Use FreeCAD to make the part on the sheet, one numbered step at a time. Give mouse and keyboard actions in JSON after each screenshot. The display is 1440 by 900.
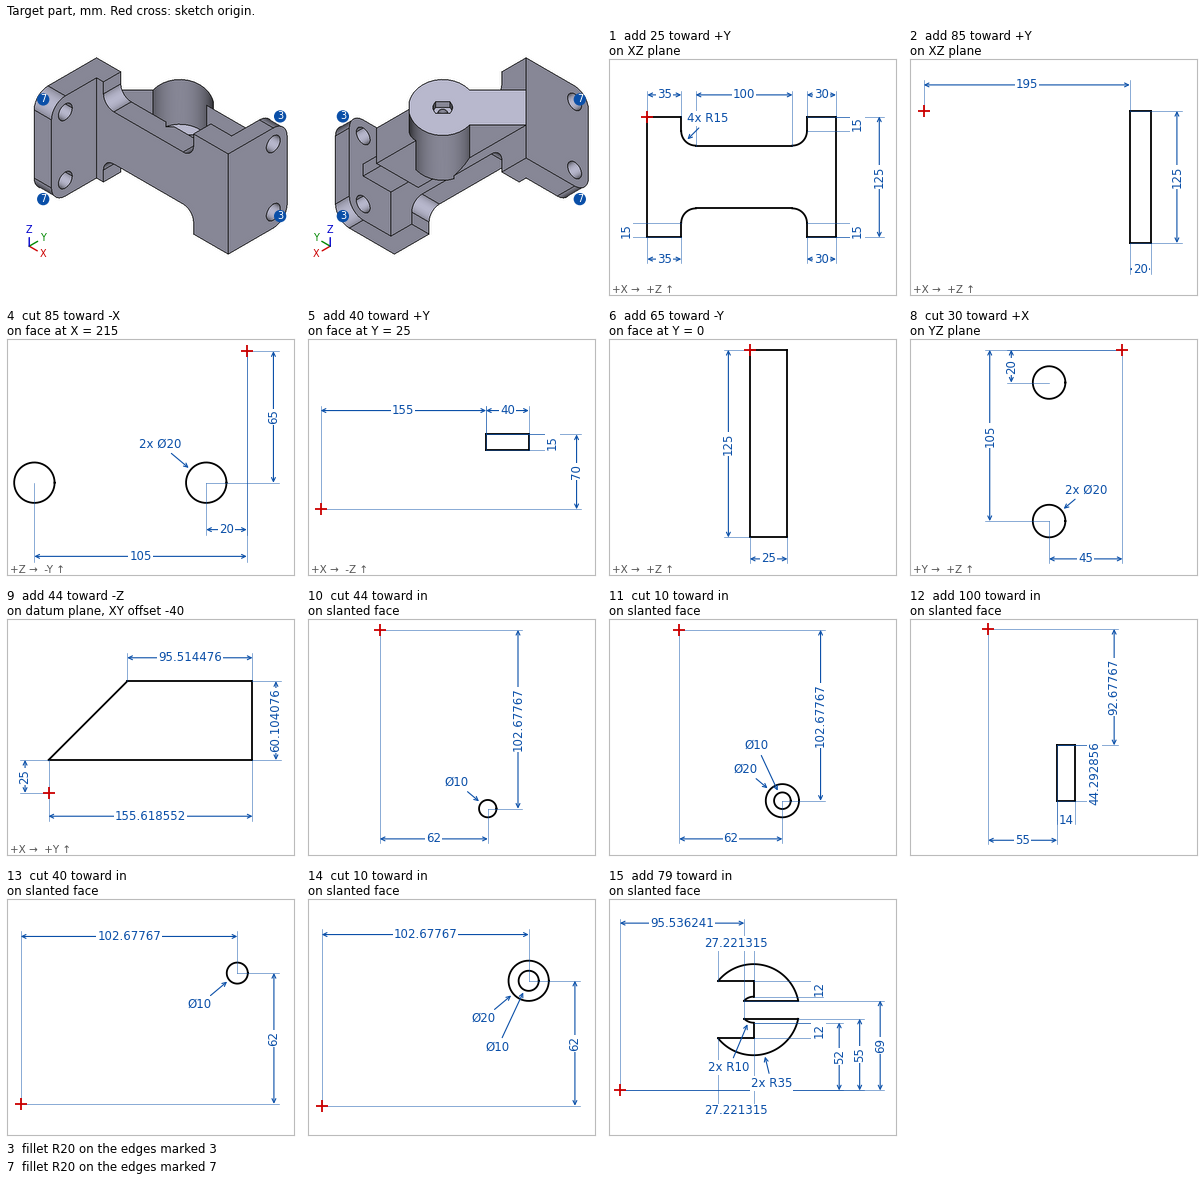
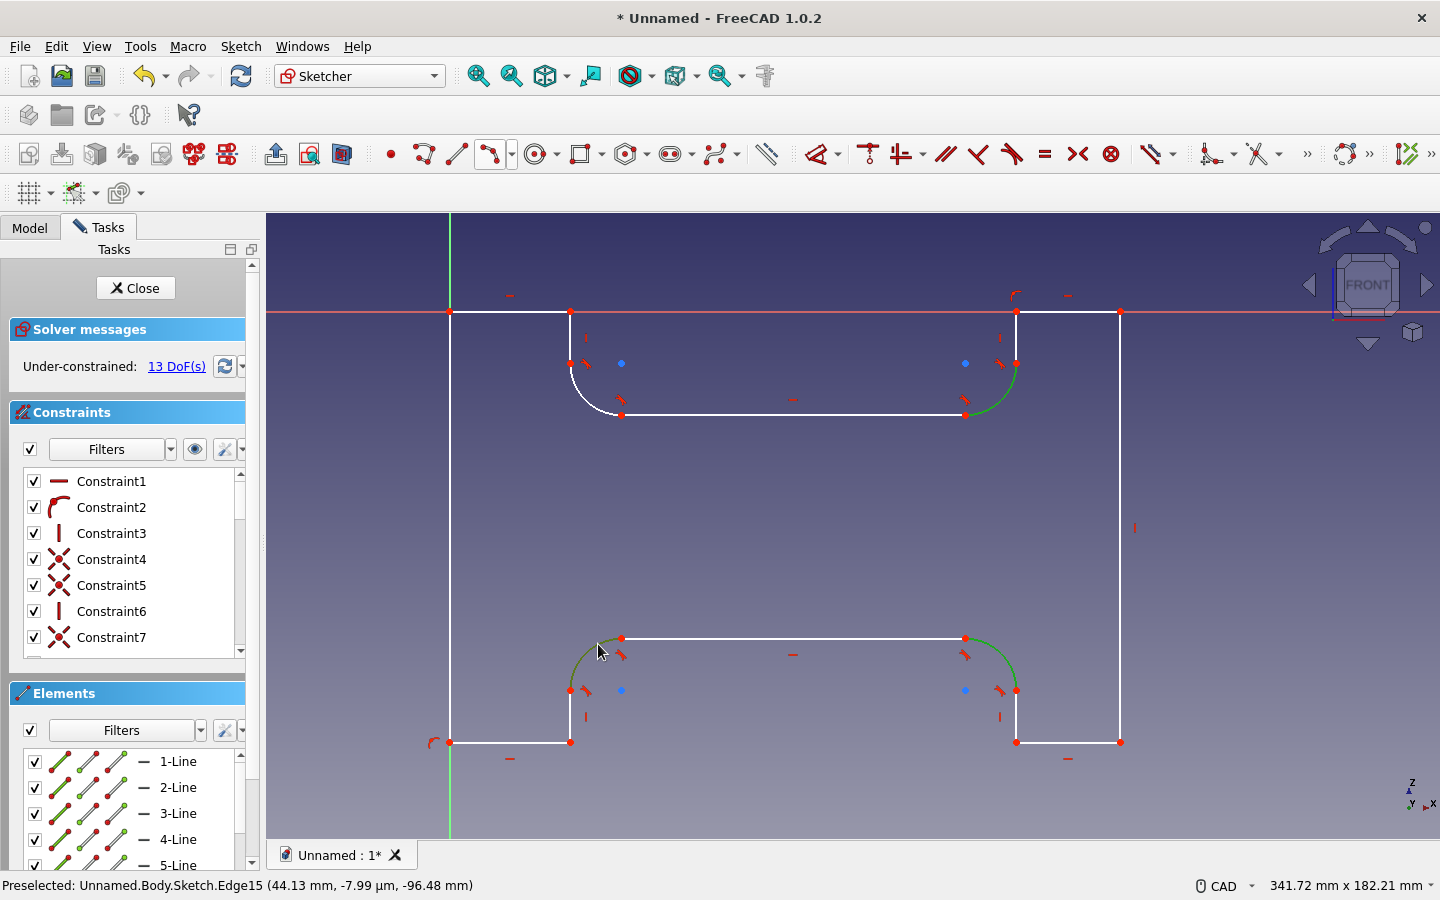
{"action": "left_click", "coordinate": [576, 387]}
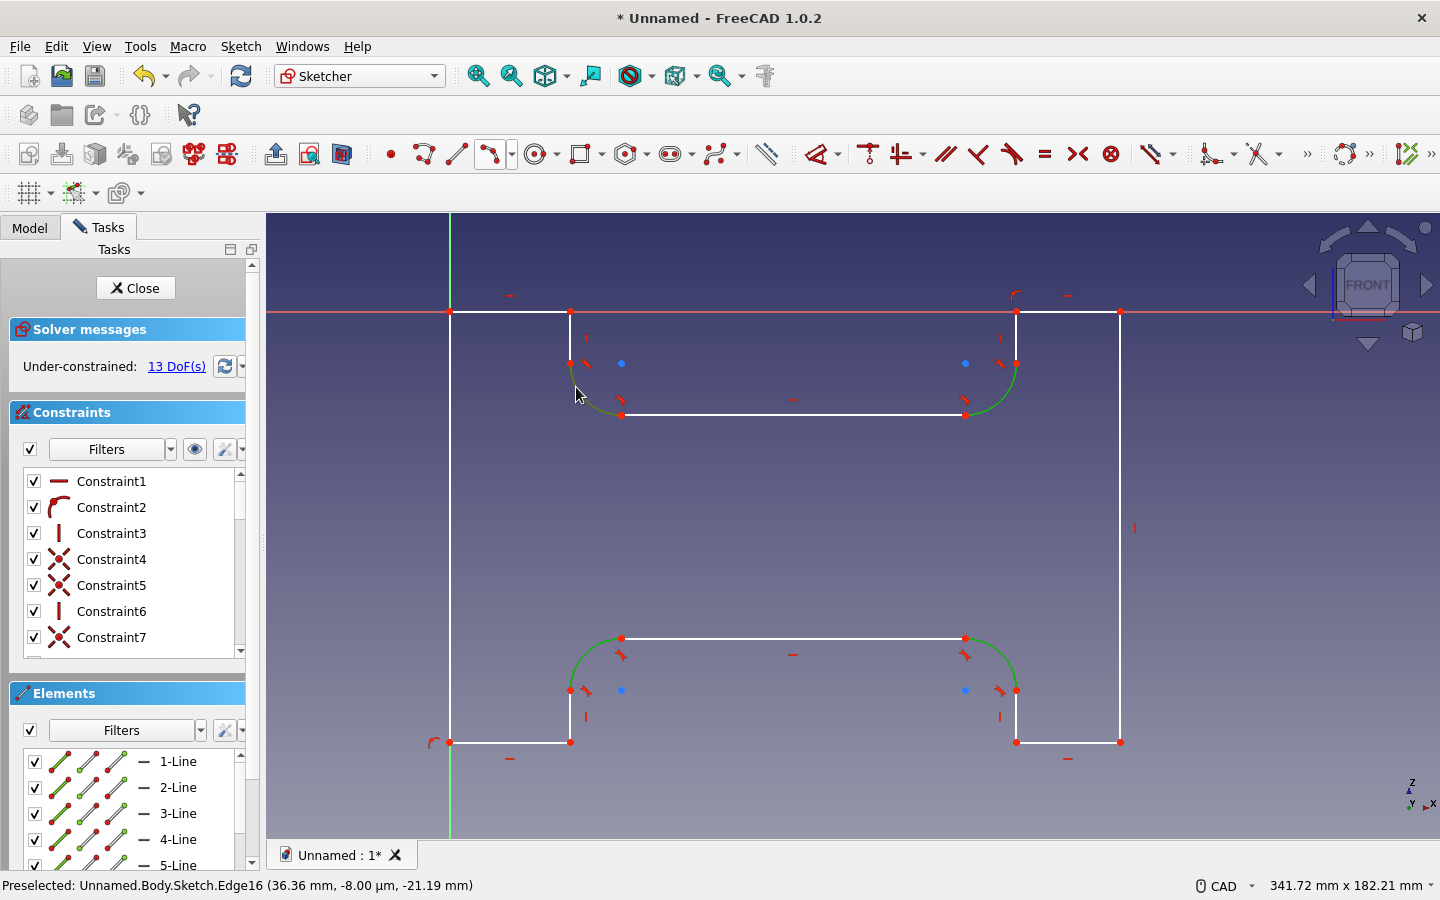
{"action": "key", "text": "e"}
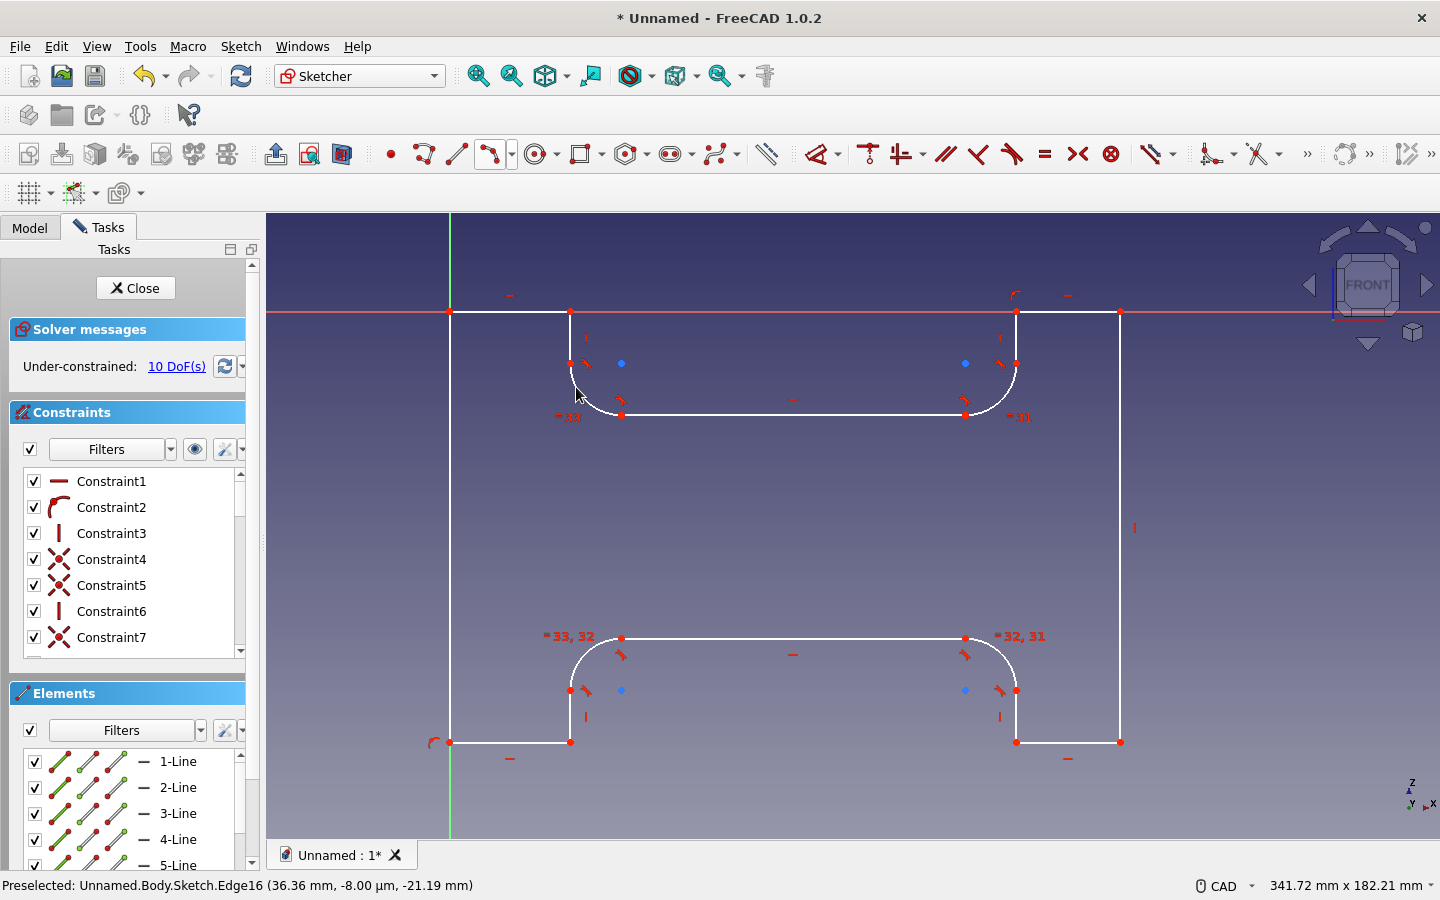
{"action": "left_click", "coordinate": [816, 154]}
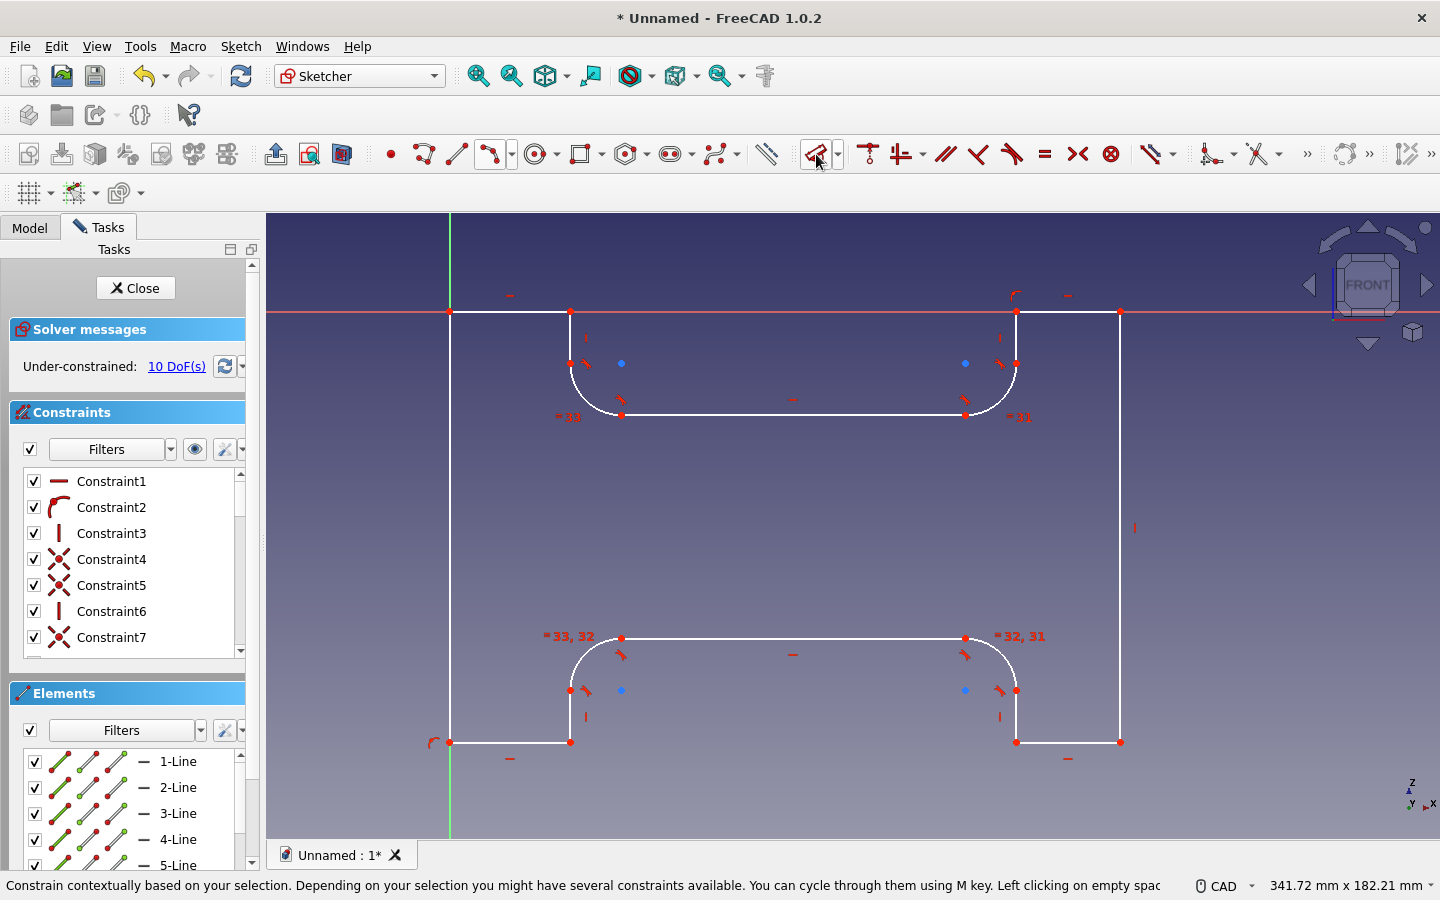
{"action": "left_click", "coordinate": [988, 410]}
{"action": "left_click", "coordinate": [1002, 439]}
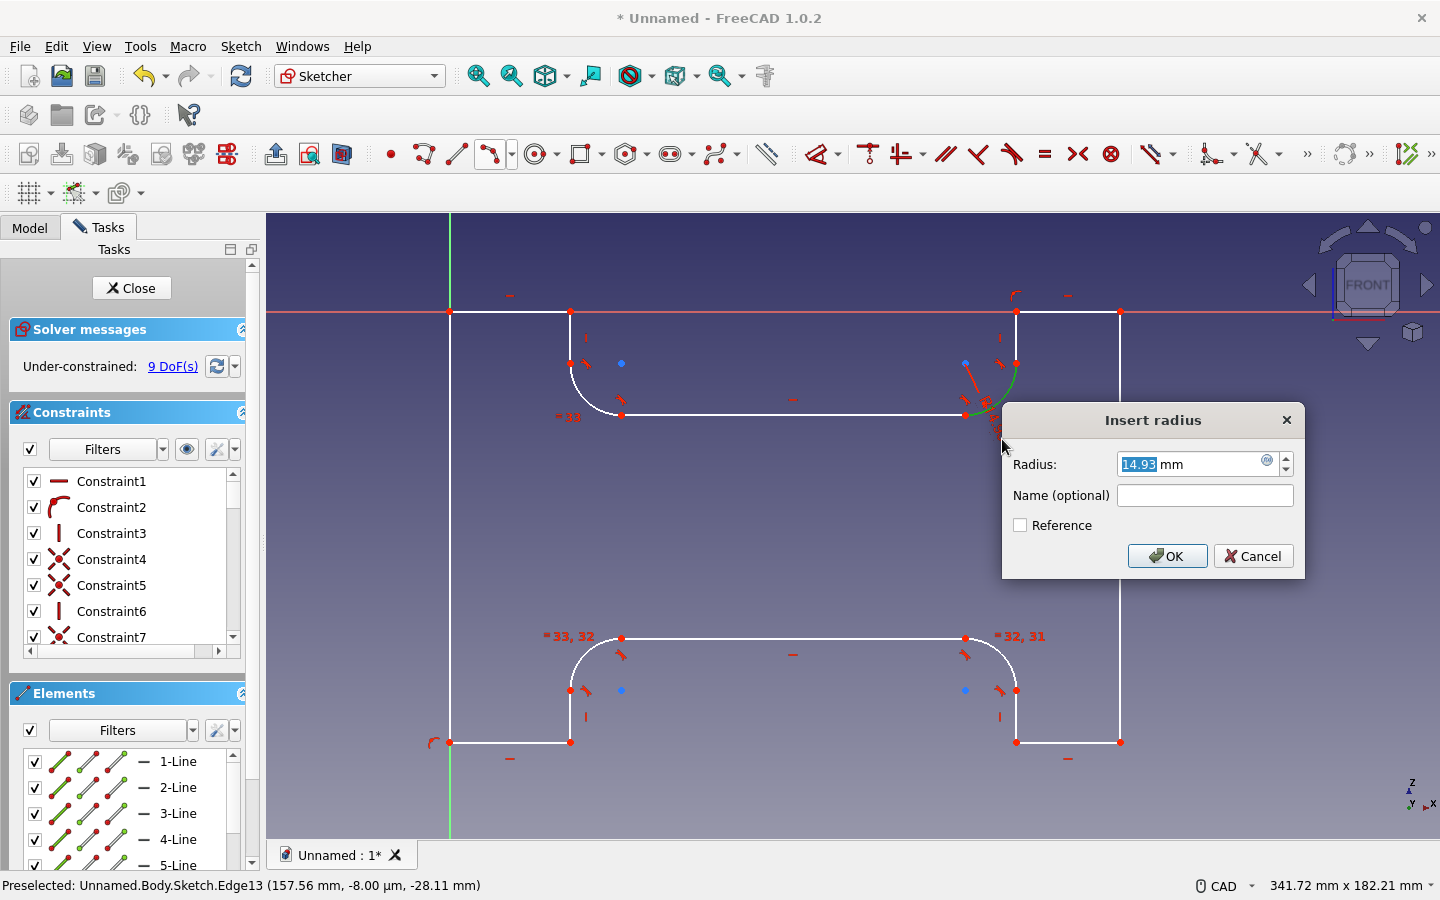
{"action": "type", "text": "15"}
{"action": "key", "text": "Return"}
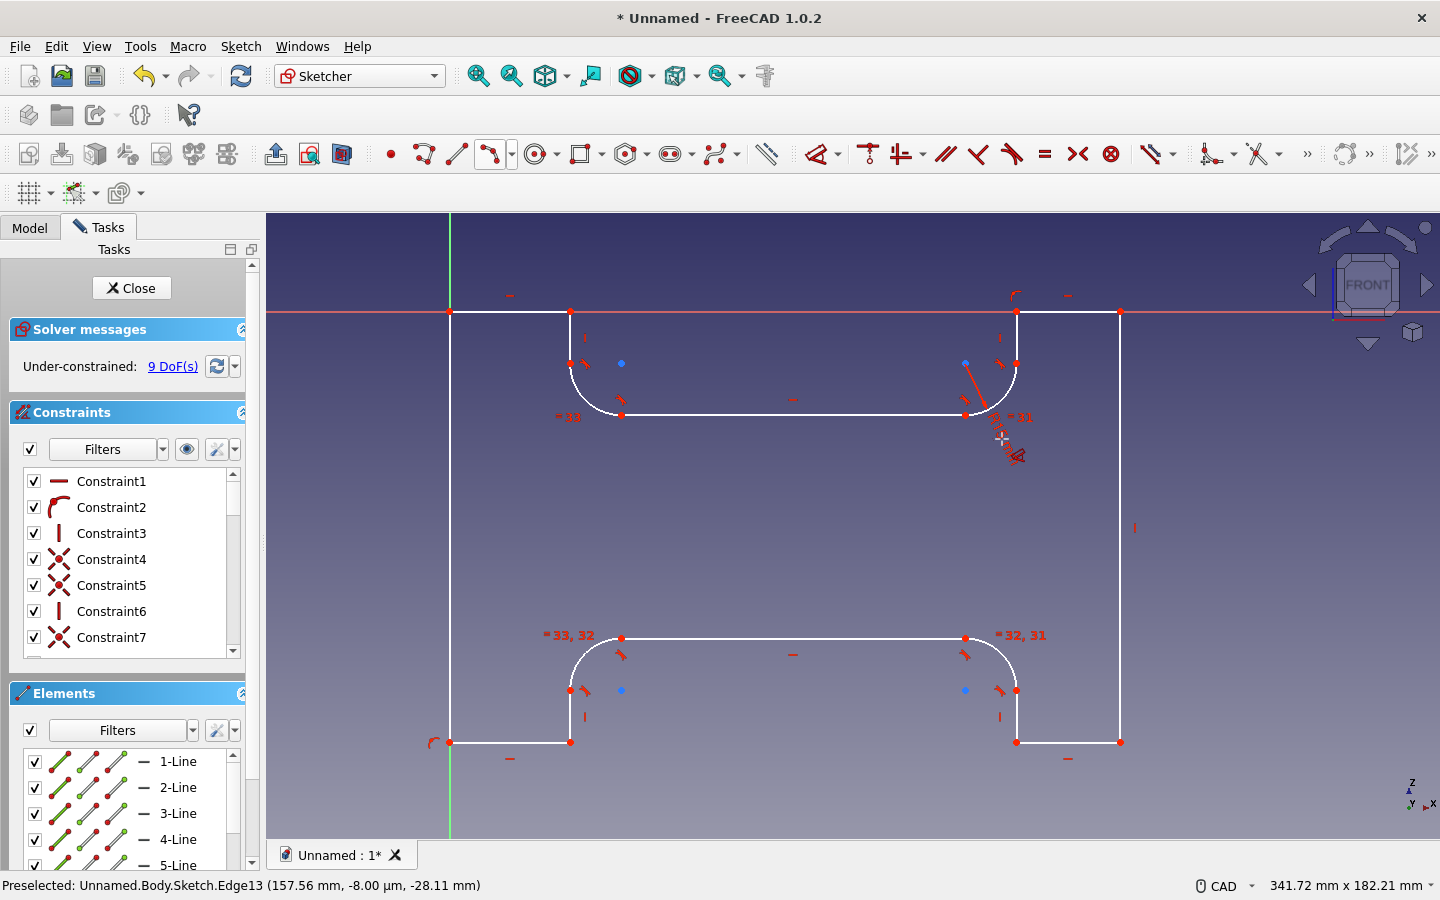
{"action": "left_click", "coordinate": [1017, 348]}
{"action": "left_click", "coordinate": [1051, 338]}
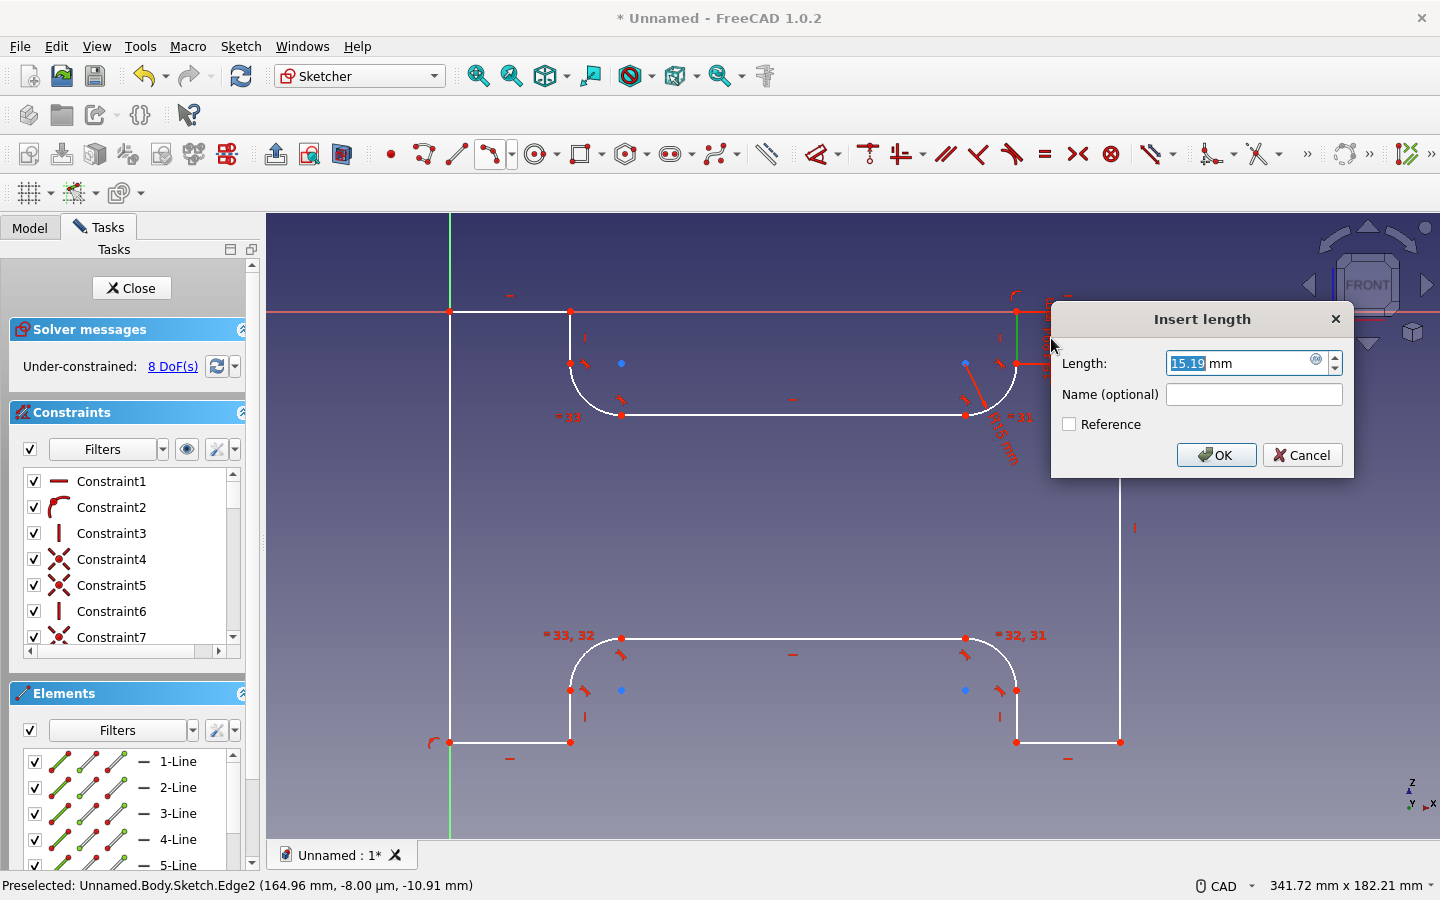
{"action": "type", "text": "15"}
{"action": "key", "text": "Return"}